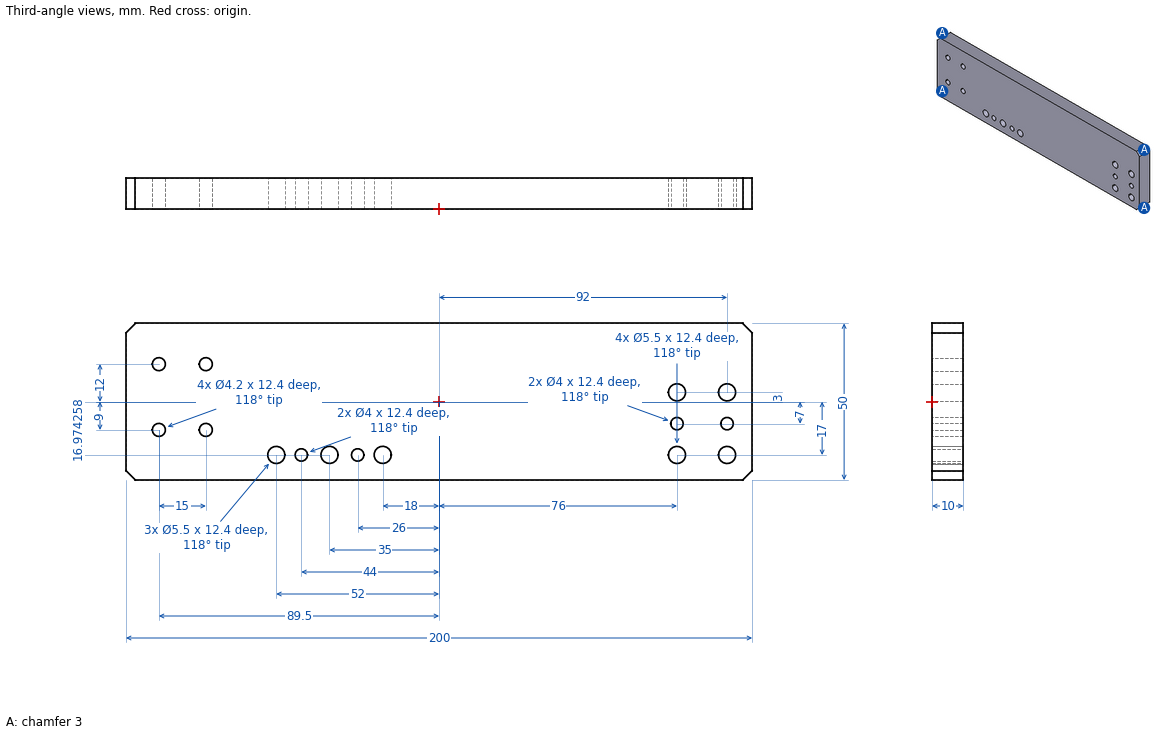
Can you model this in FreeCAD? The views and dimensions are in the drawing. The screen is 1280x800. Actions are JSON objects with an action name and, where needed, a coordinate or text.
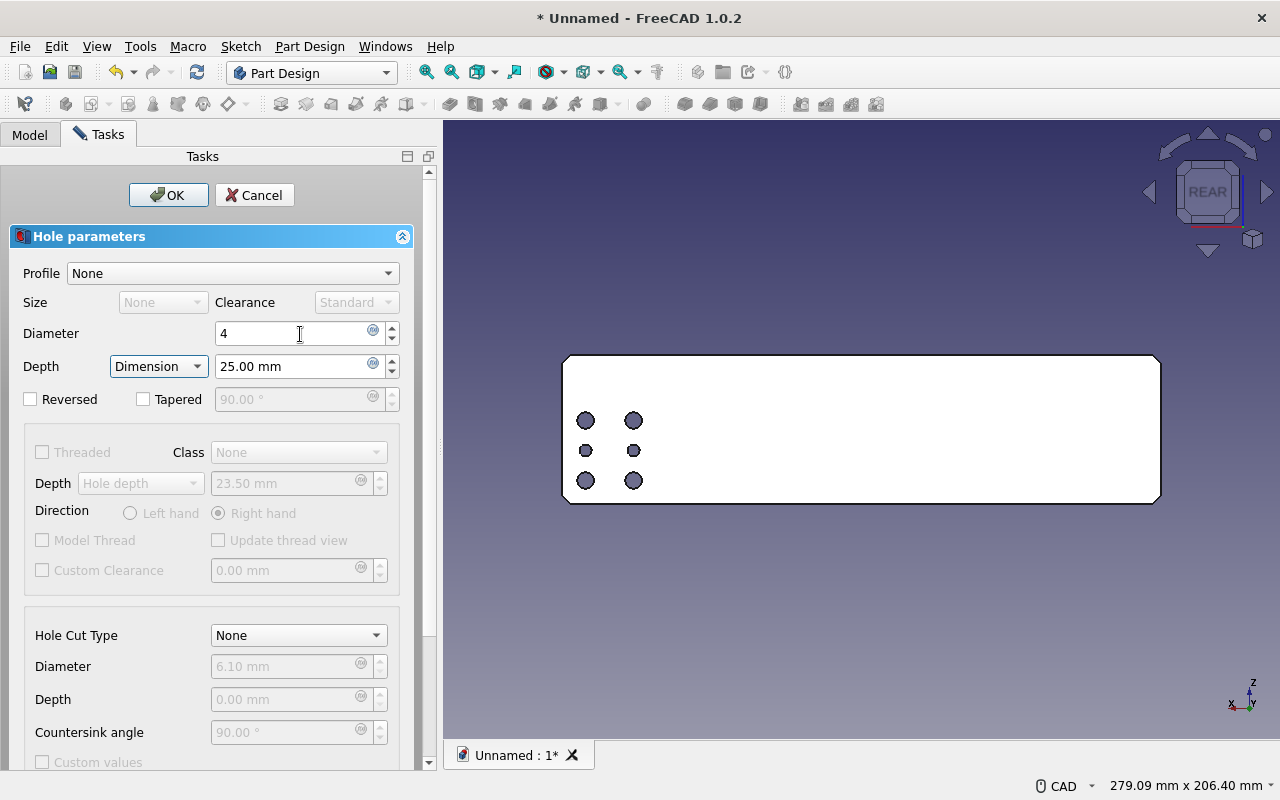
{"action": "triple_click", "coordinate": [300, 366]}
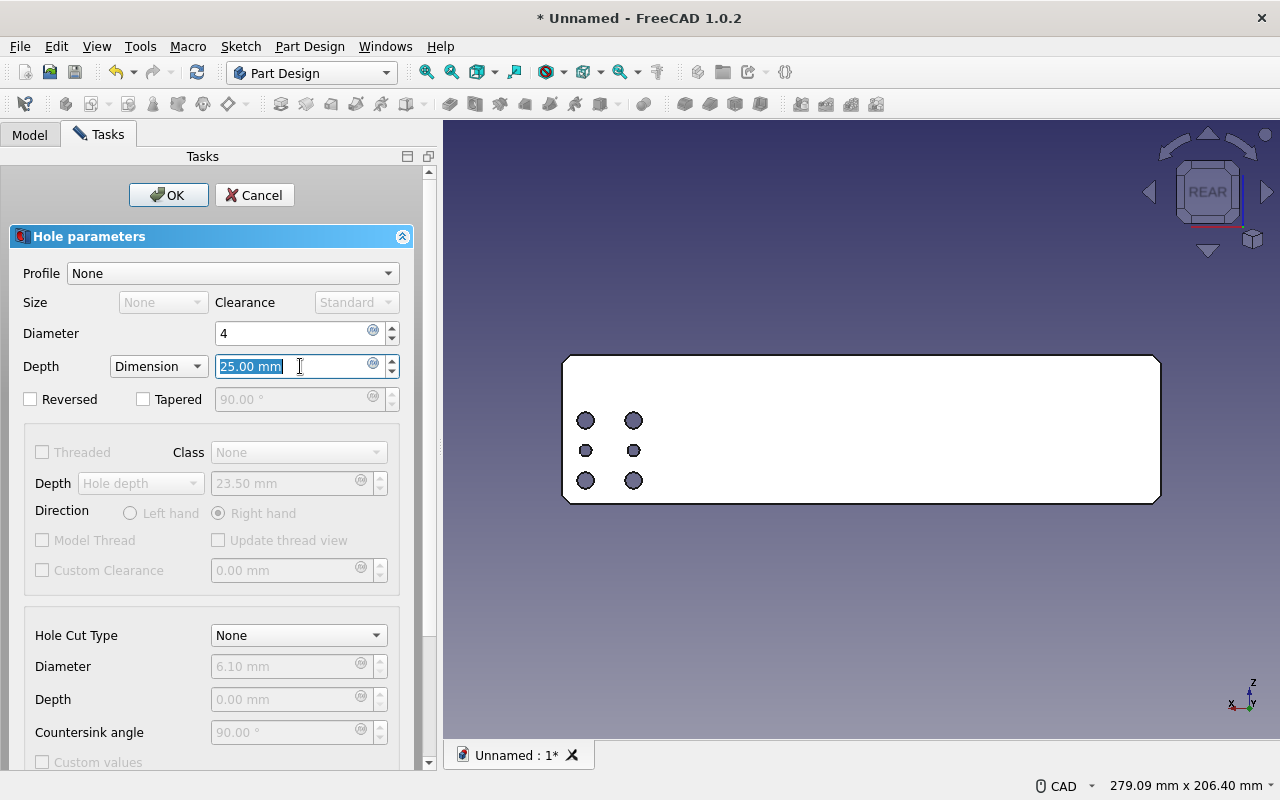
{"action": "type", "text": "12.4"}
{"action": "key", "text": "Tab"}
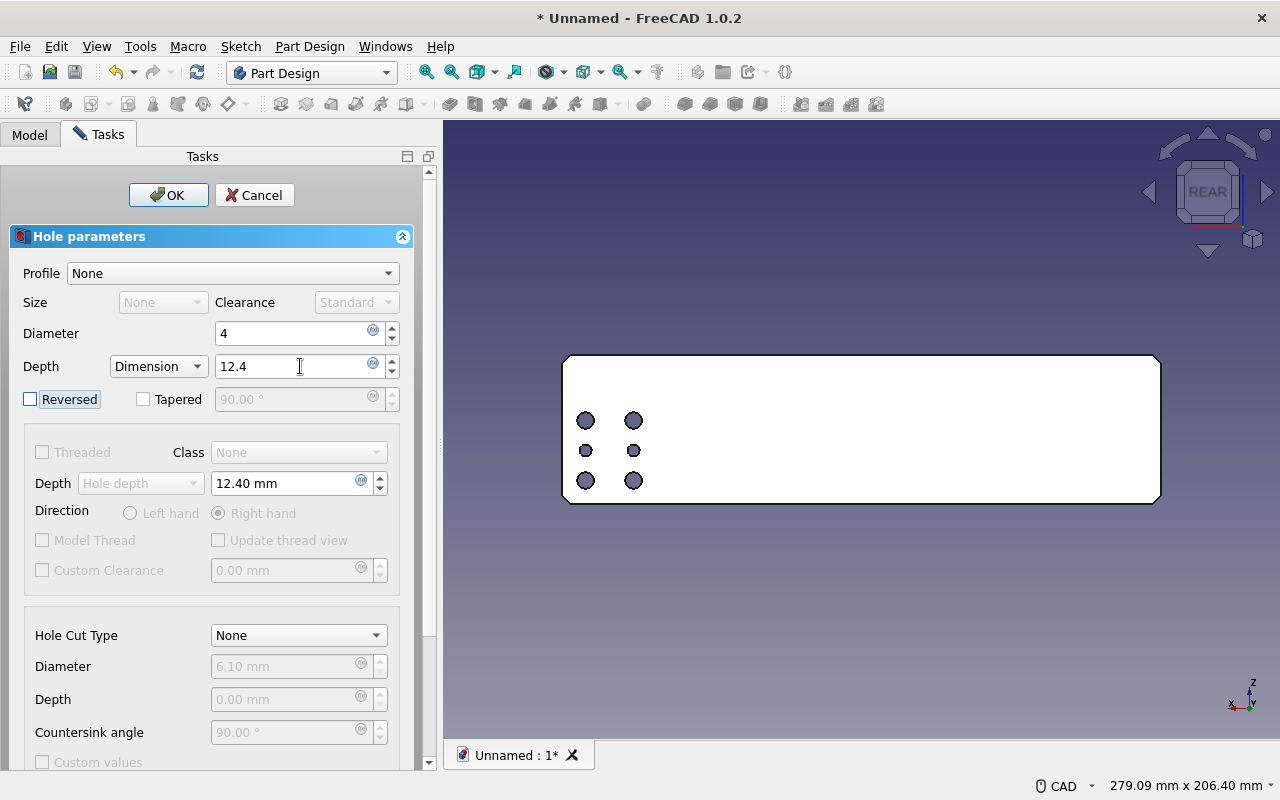
{"action": "left_click", "coordinate": [169, 195]}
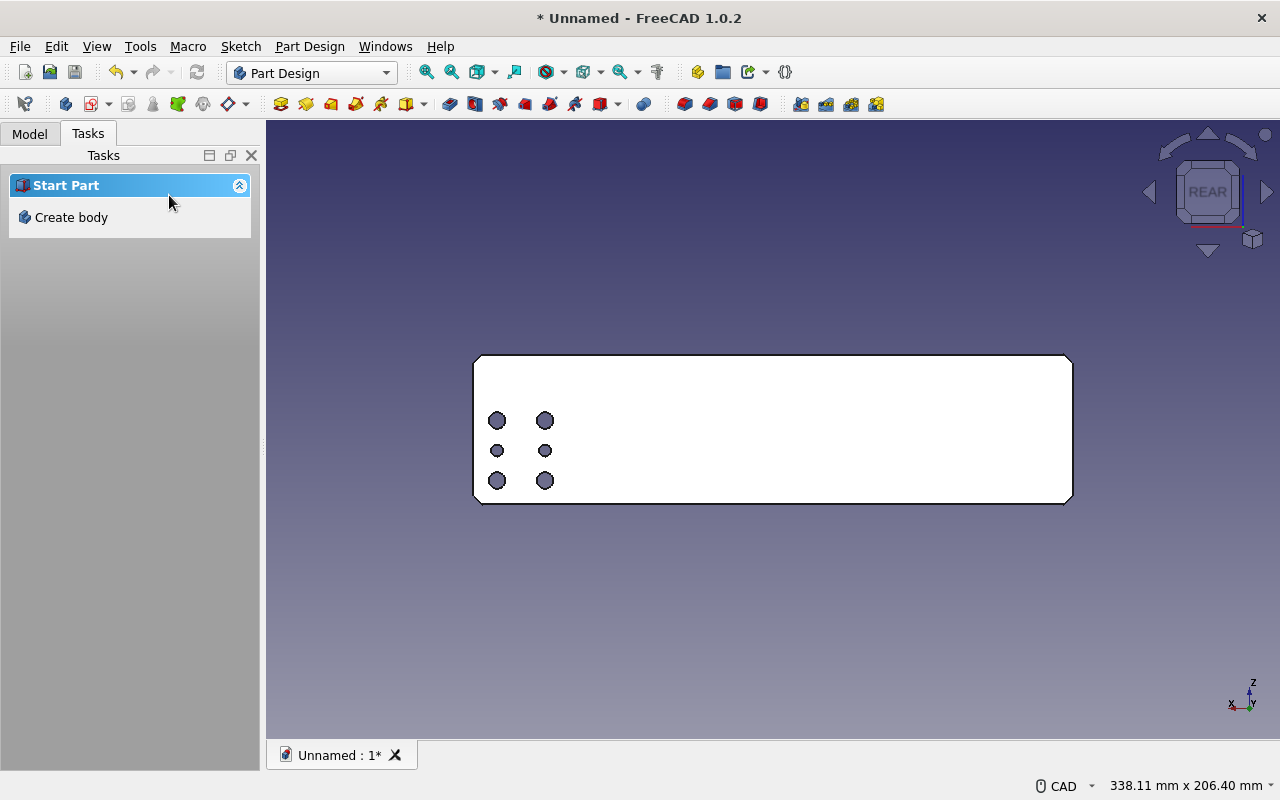
{"action": "left_click", "coordinate": [687, 429]}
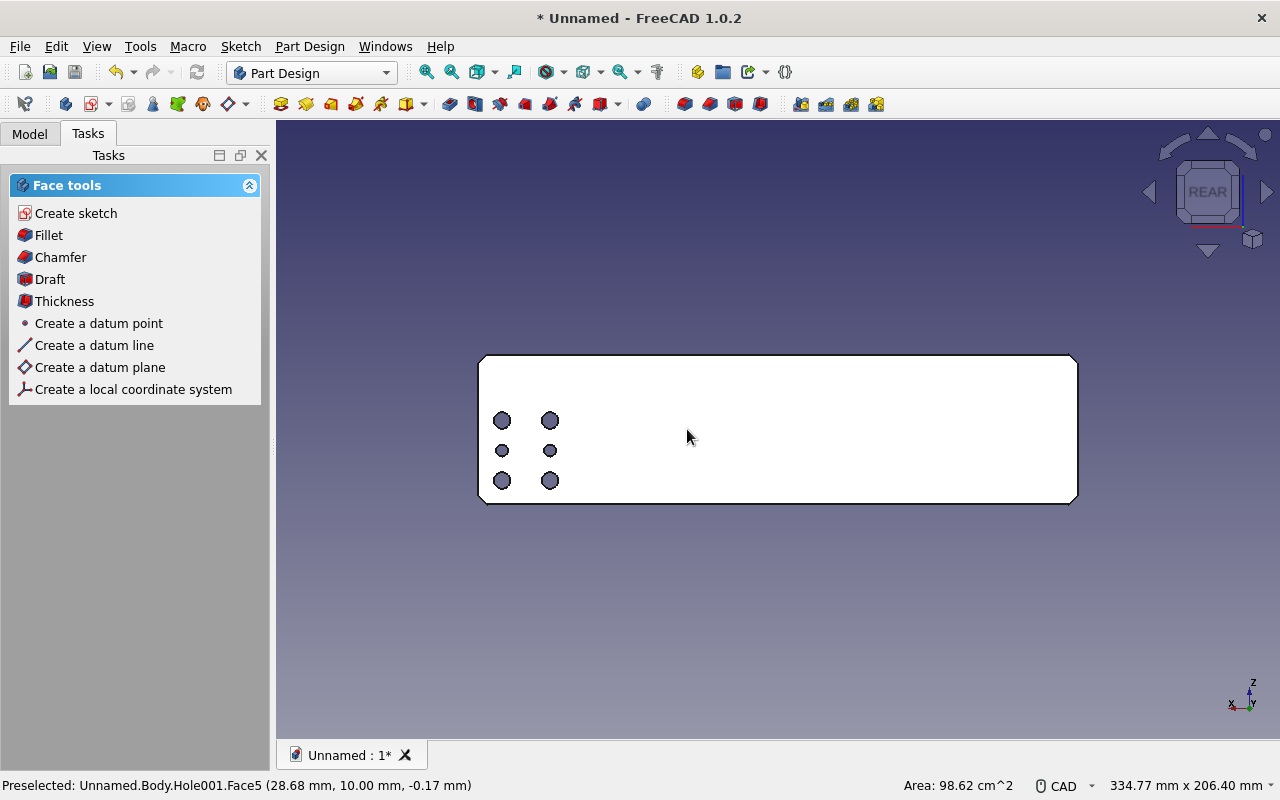
{"action": "left_click", "coordinate": [90, 104]}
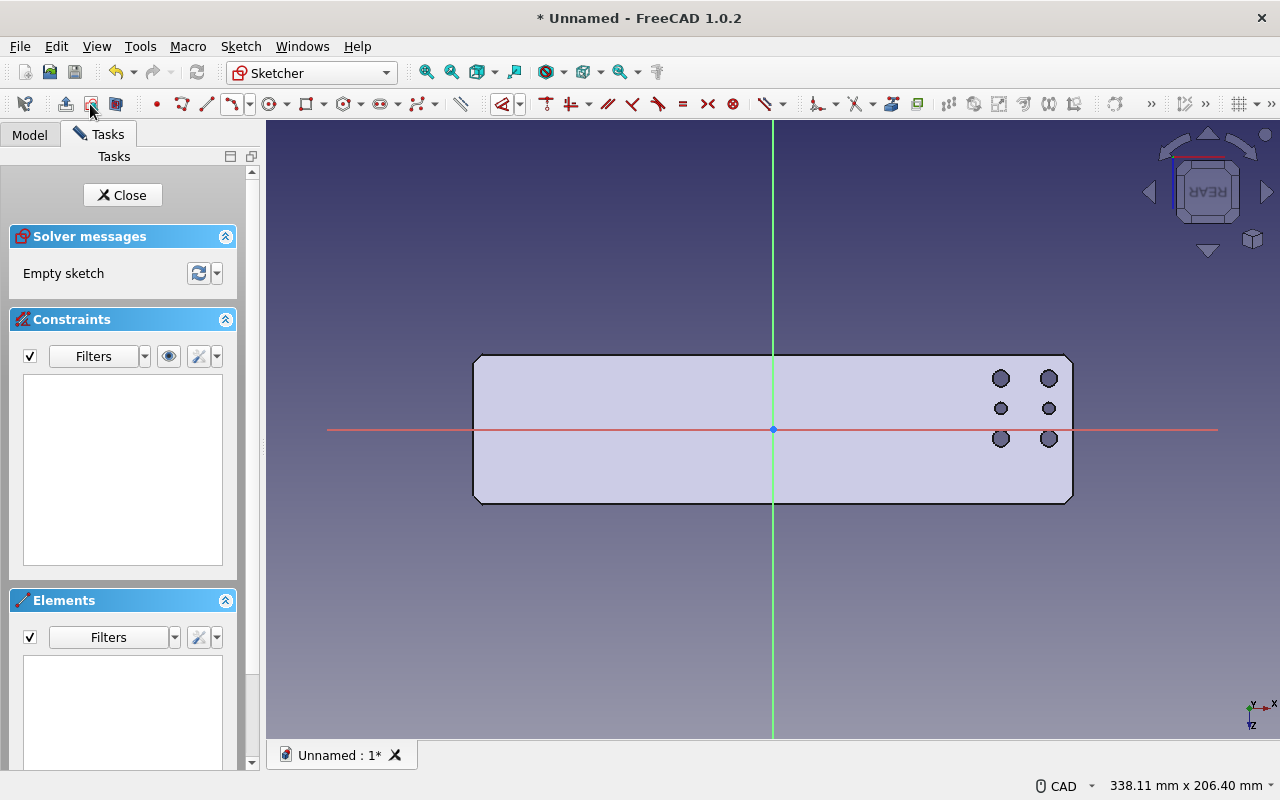
{"action": "scroll", "coordinate": [482, 435], "scroll_direction": "up", "scroll_amount": 8}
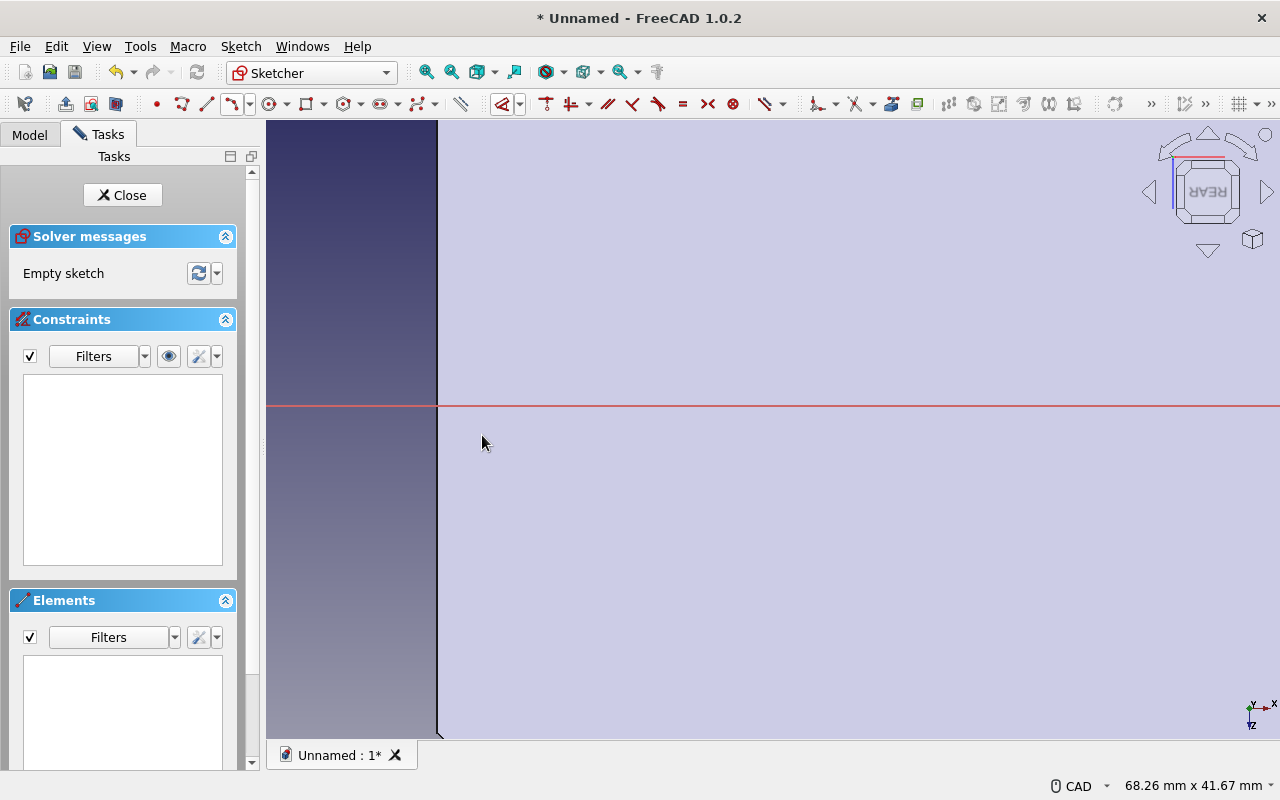
{"action": "key", "text": "g c"}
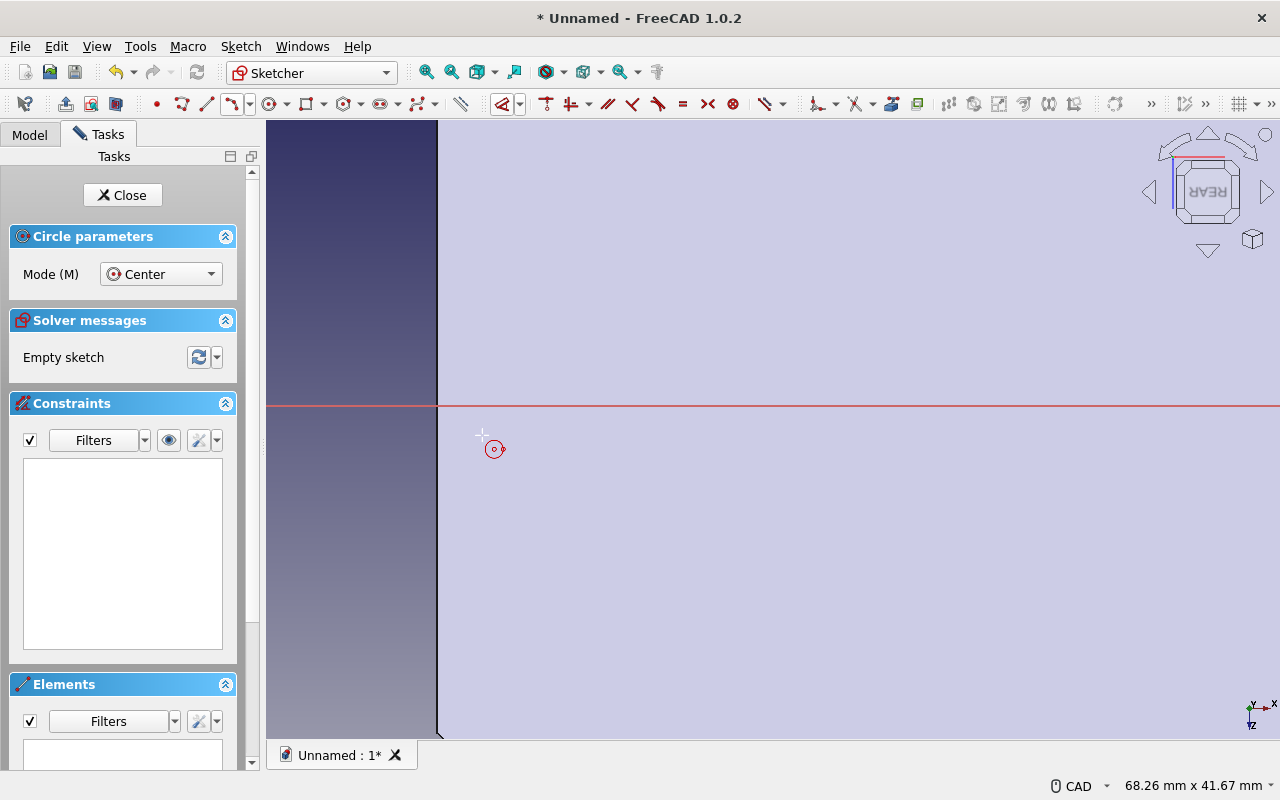
{"action": "left_click", "coordinate": [593, 272]}
{"action": "left_click", "coordinate": [615, 250]}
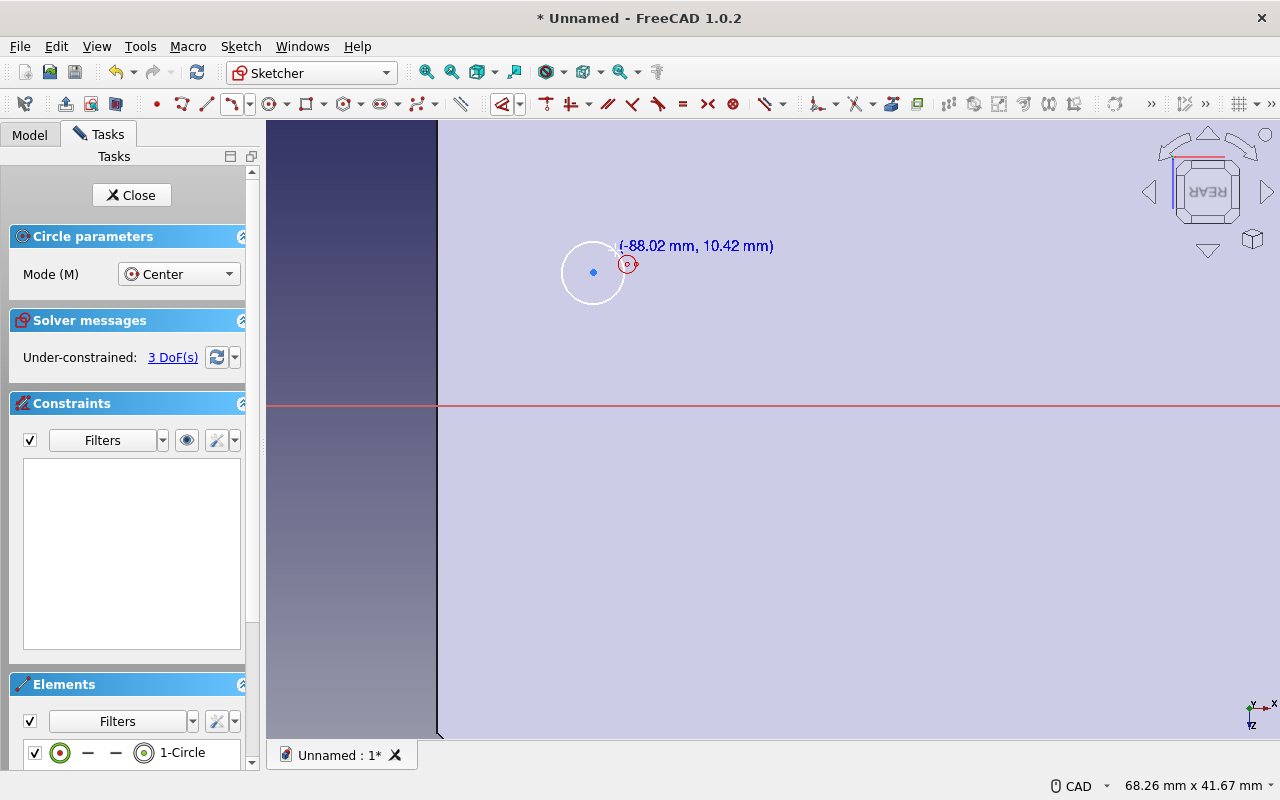
{"action": "left_click", "coordinate": [816, 272]}
{"action": "left_click", "coordinate": [838, 250]}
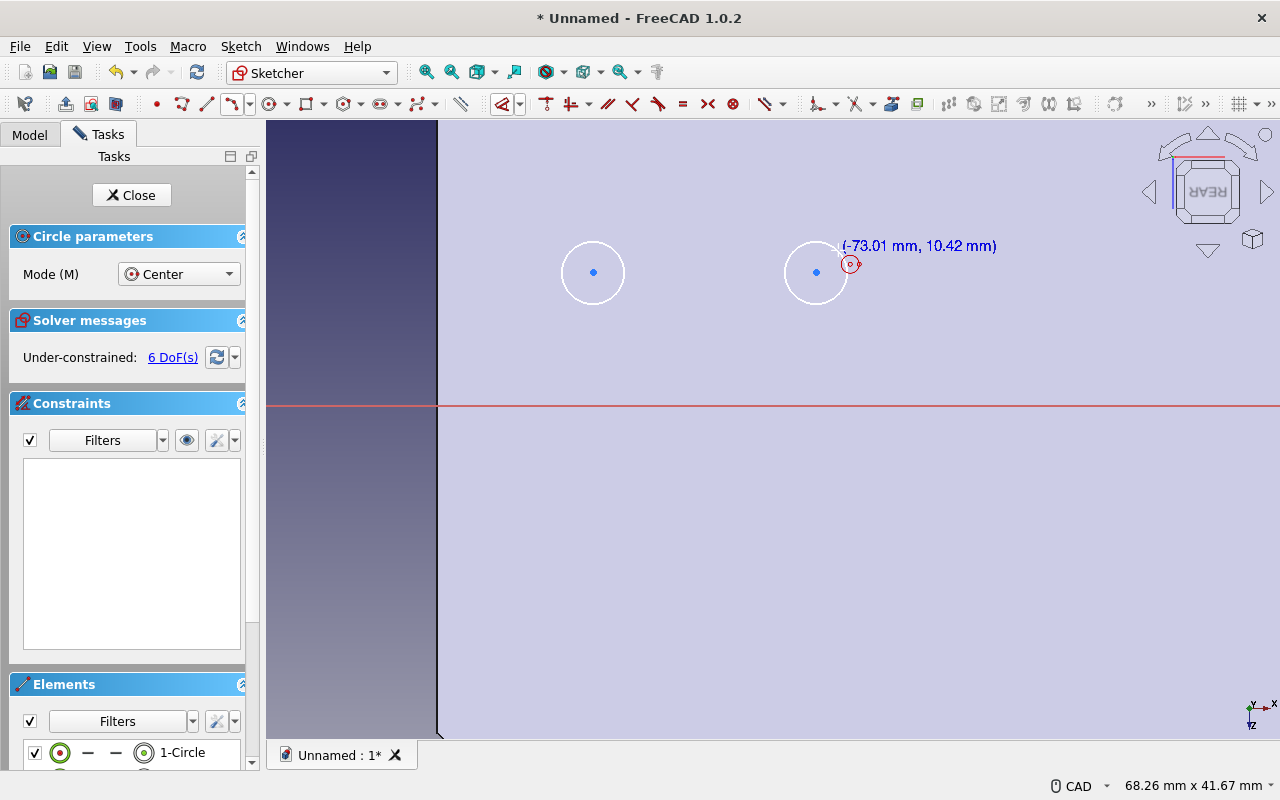
{"action": "left_click", "coordinate": [593, 584]}
{"action": "left_click", "coordinate": [615, 562]}